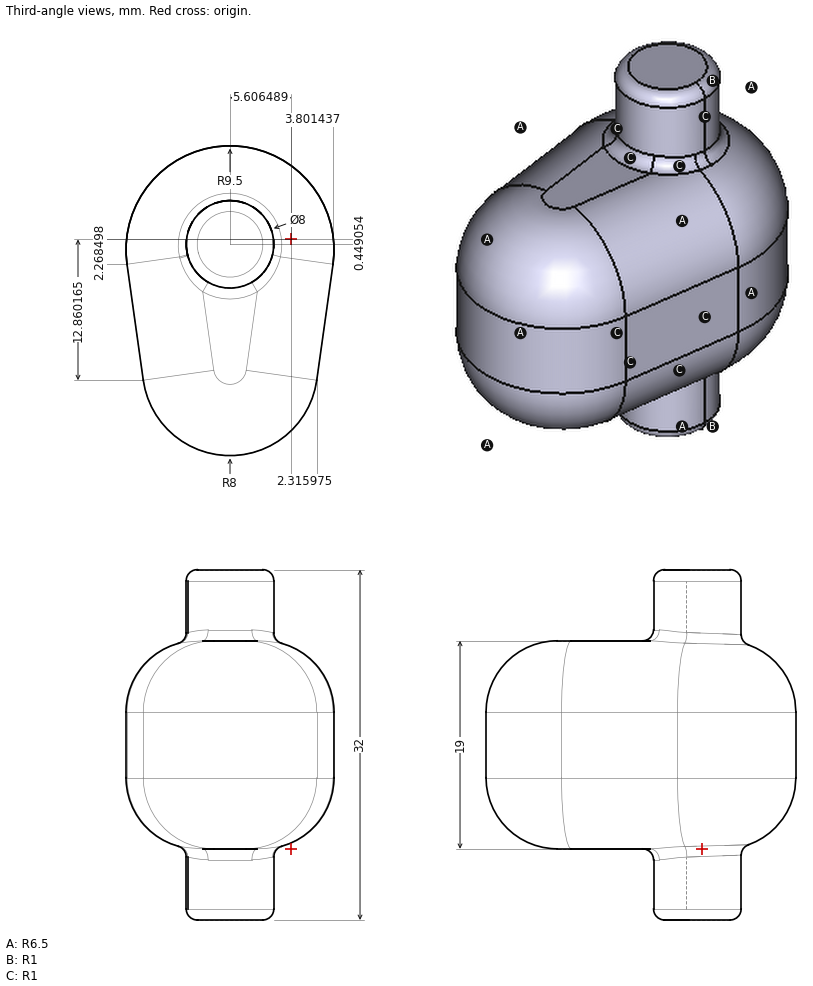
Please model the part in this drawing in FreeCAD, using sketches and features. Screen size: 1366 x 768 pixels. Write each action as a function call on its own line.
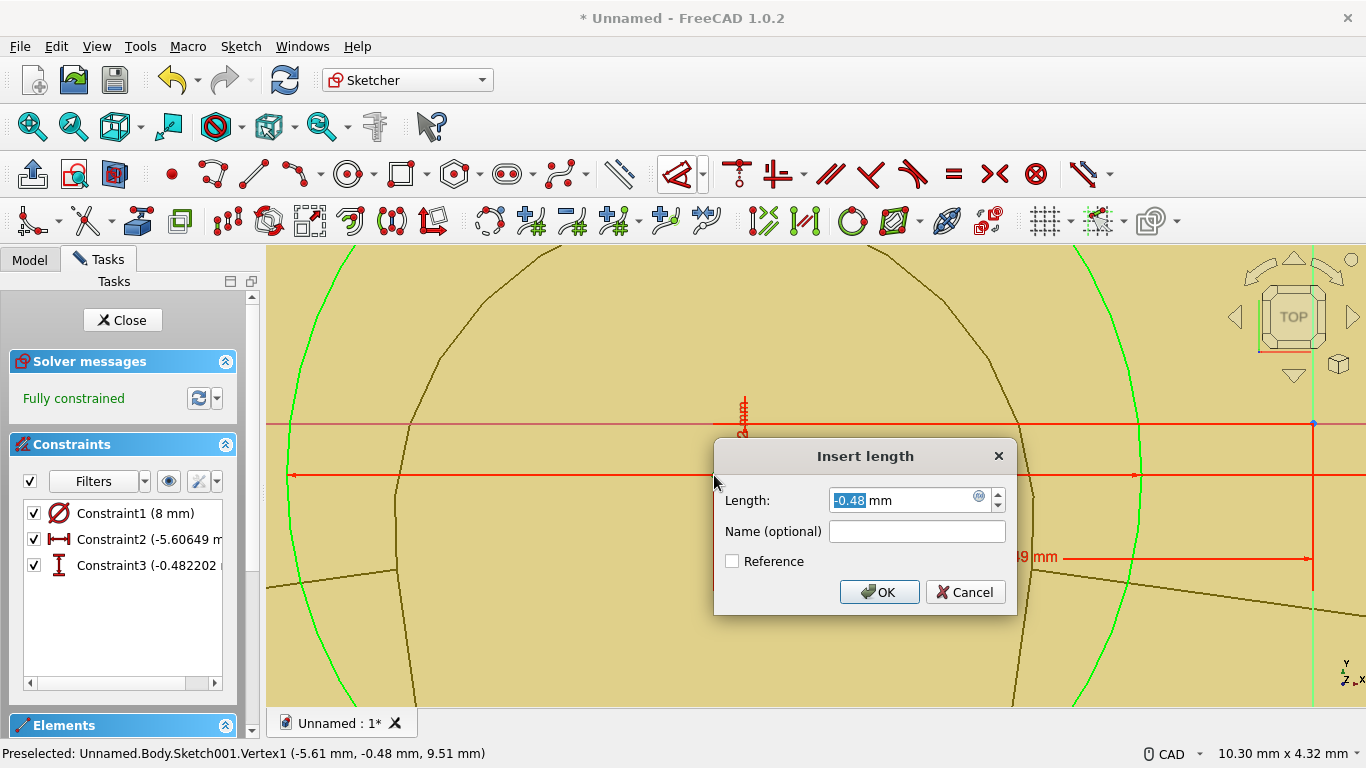
text(-0.449054)
key(Return)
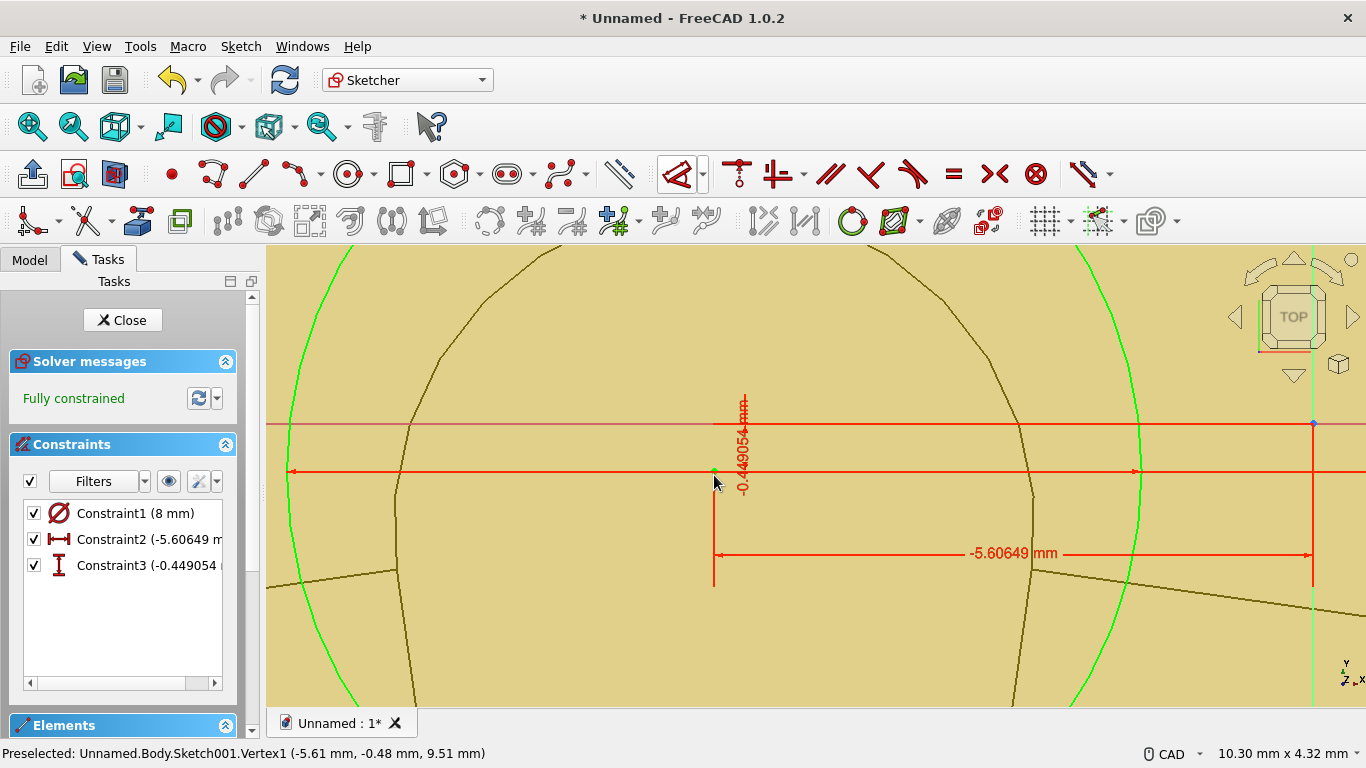
click(123, 320)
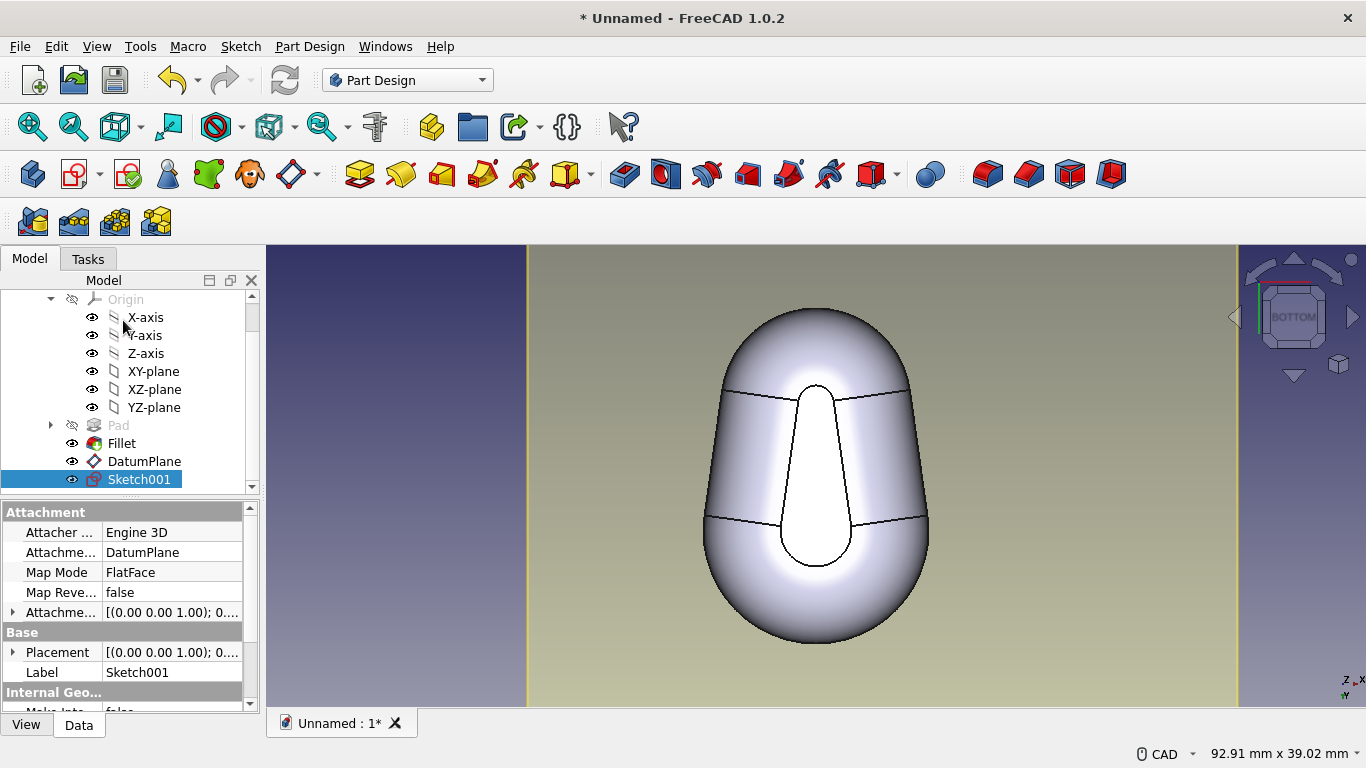
click(360, 174)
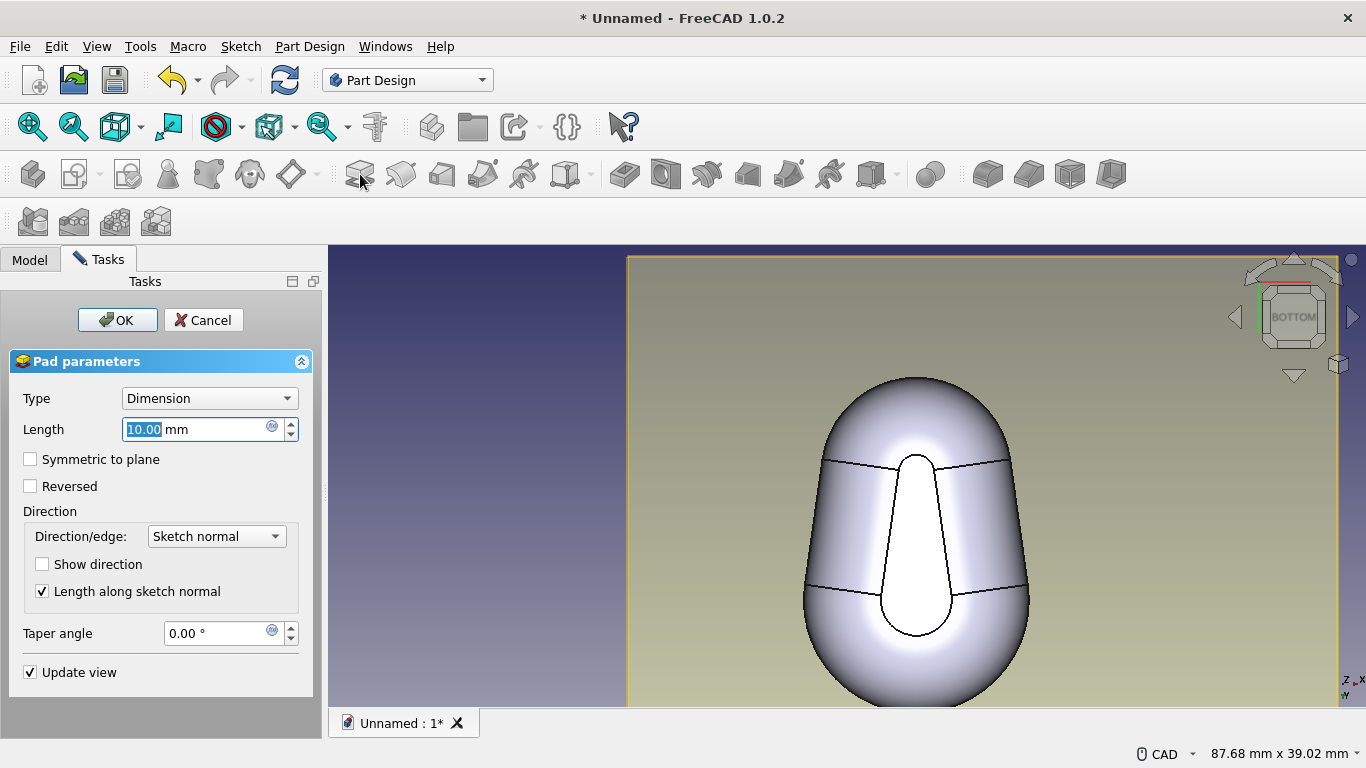
text(32)
key(Tab)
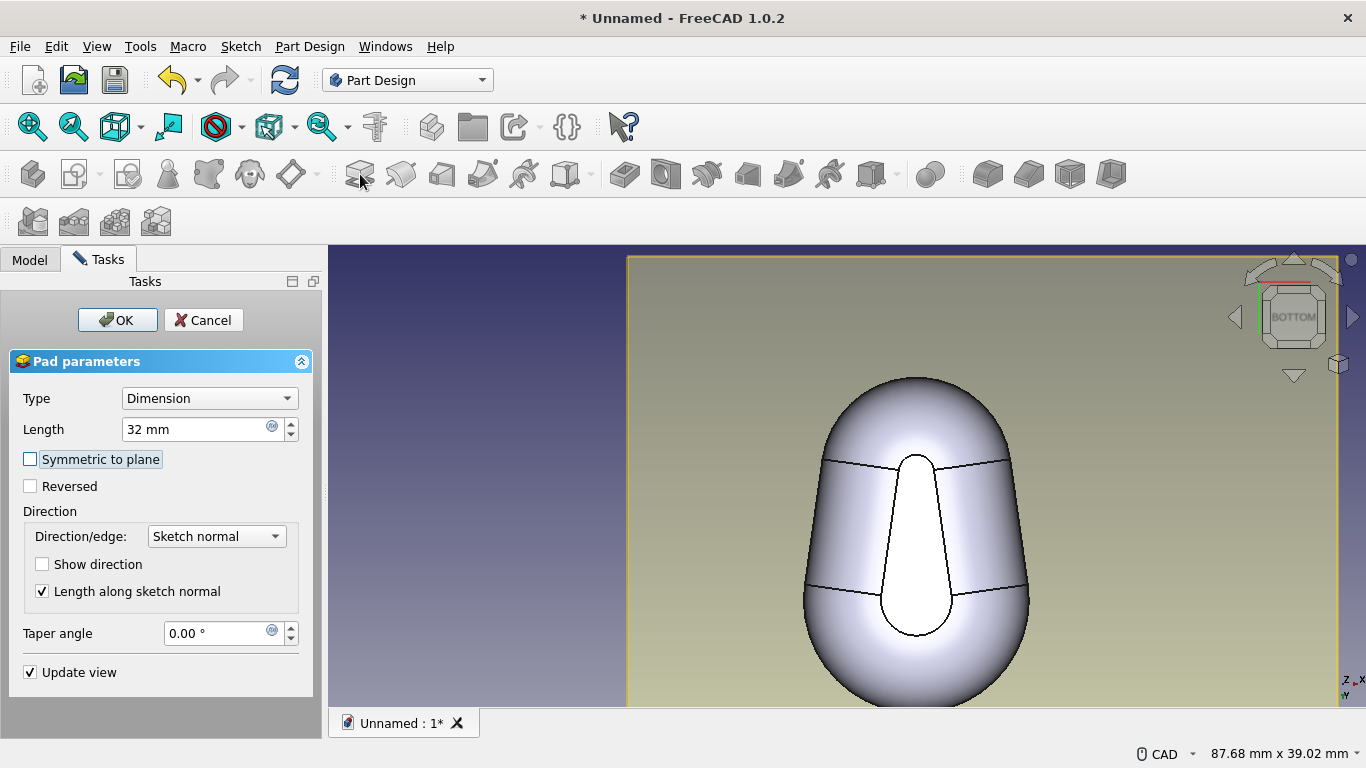
click(31, 459)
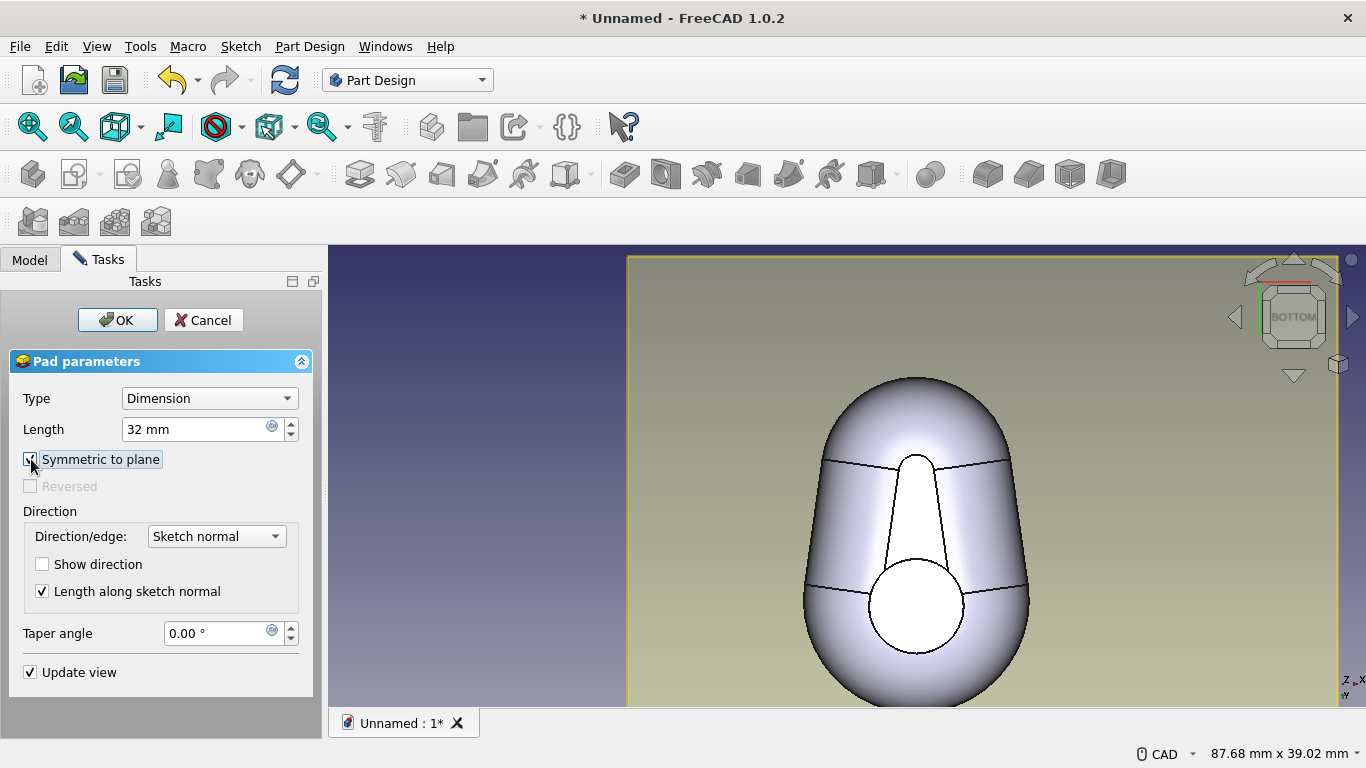
click(118, 320)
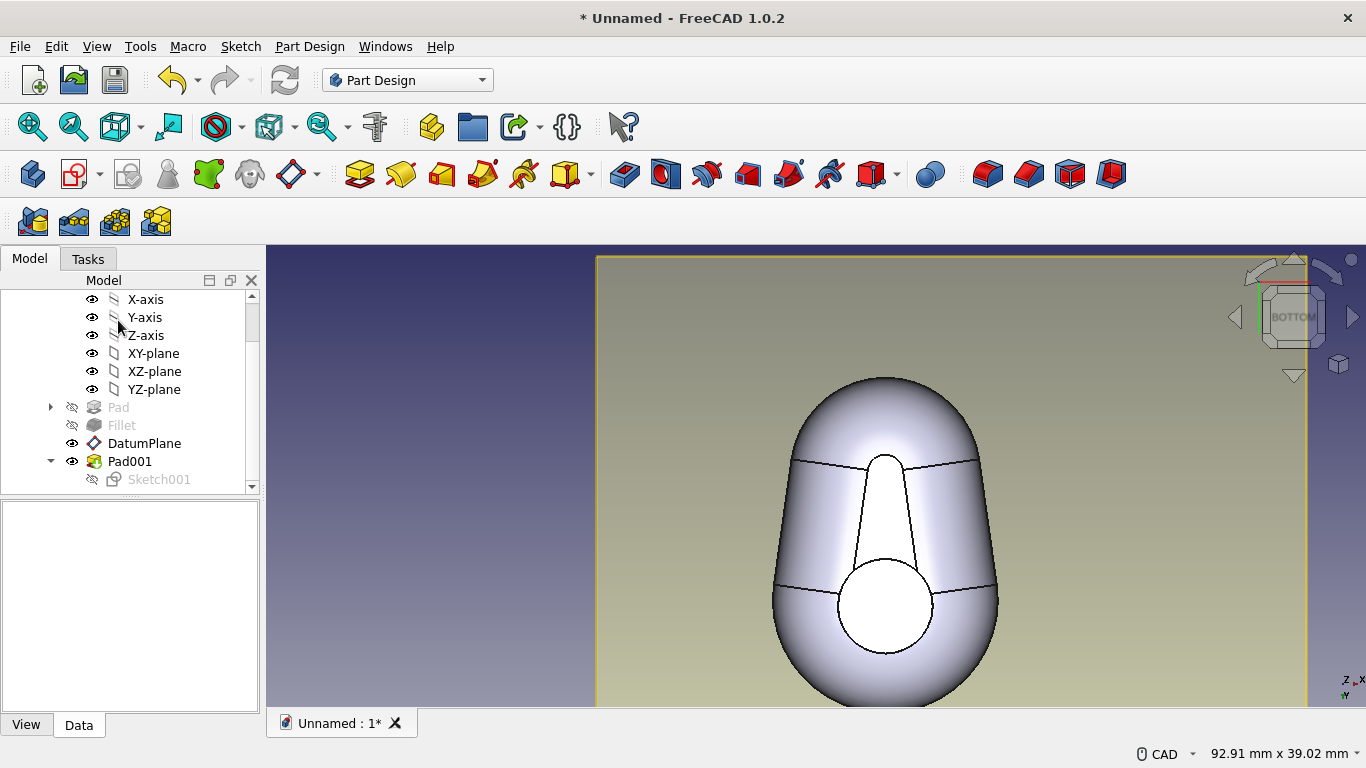
click(117, 443)
key(space)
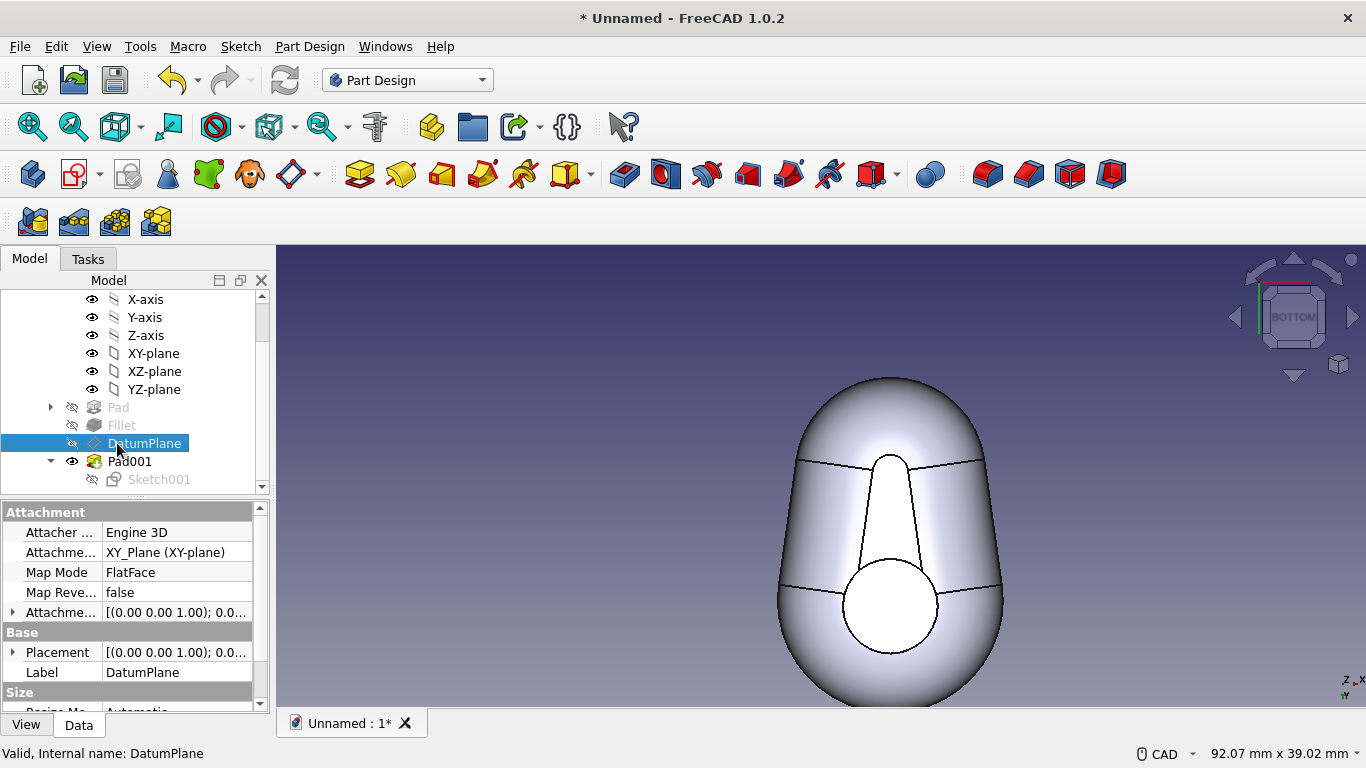
key(v)
key(f)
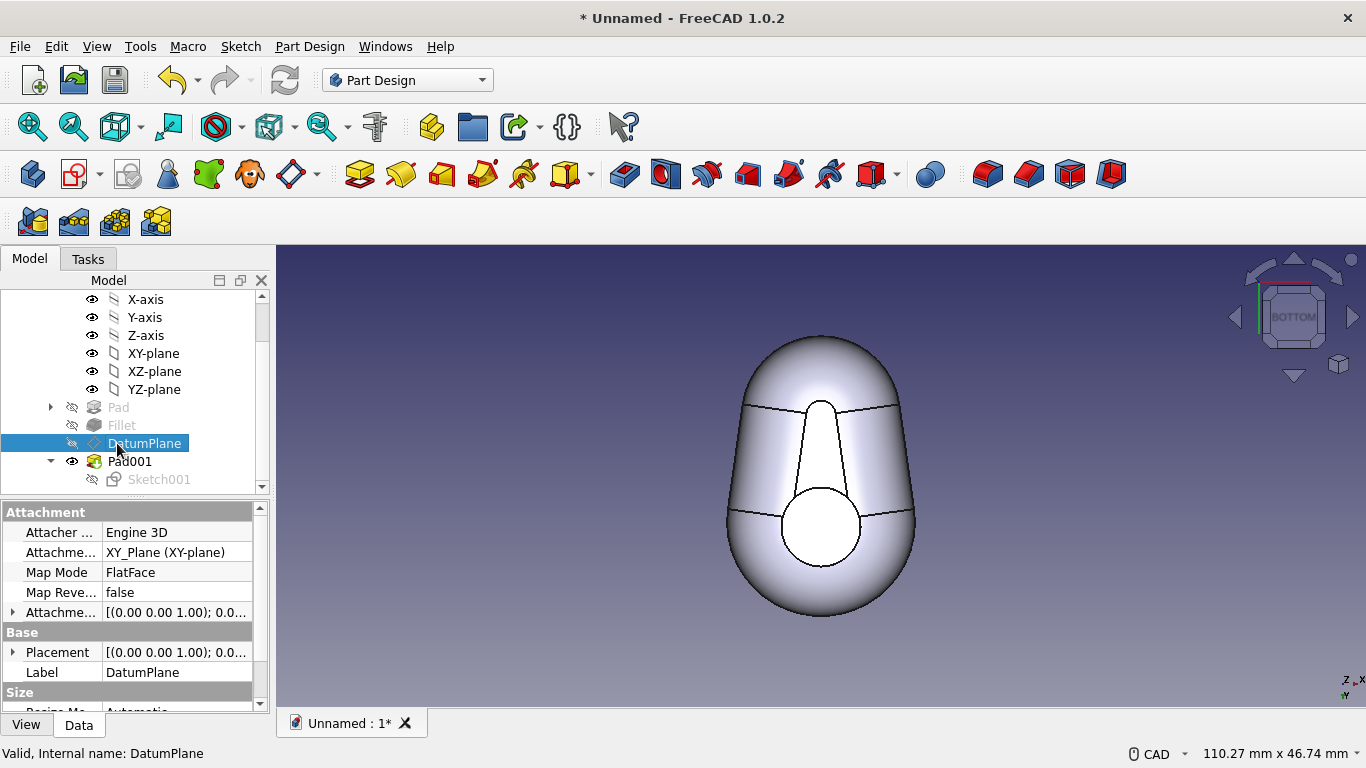
click(781, 526)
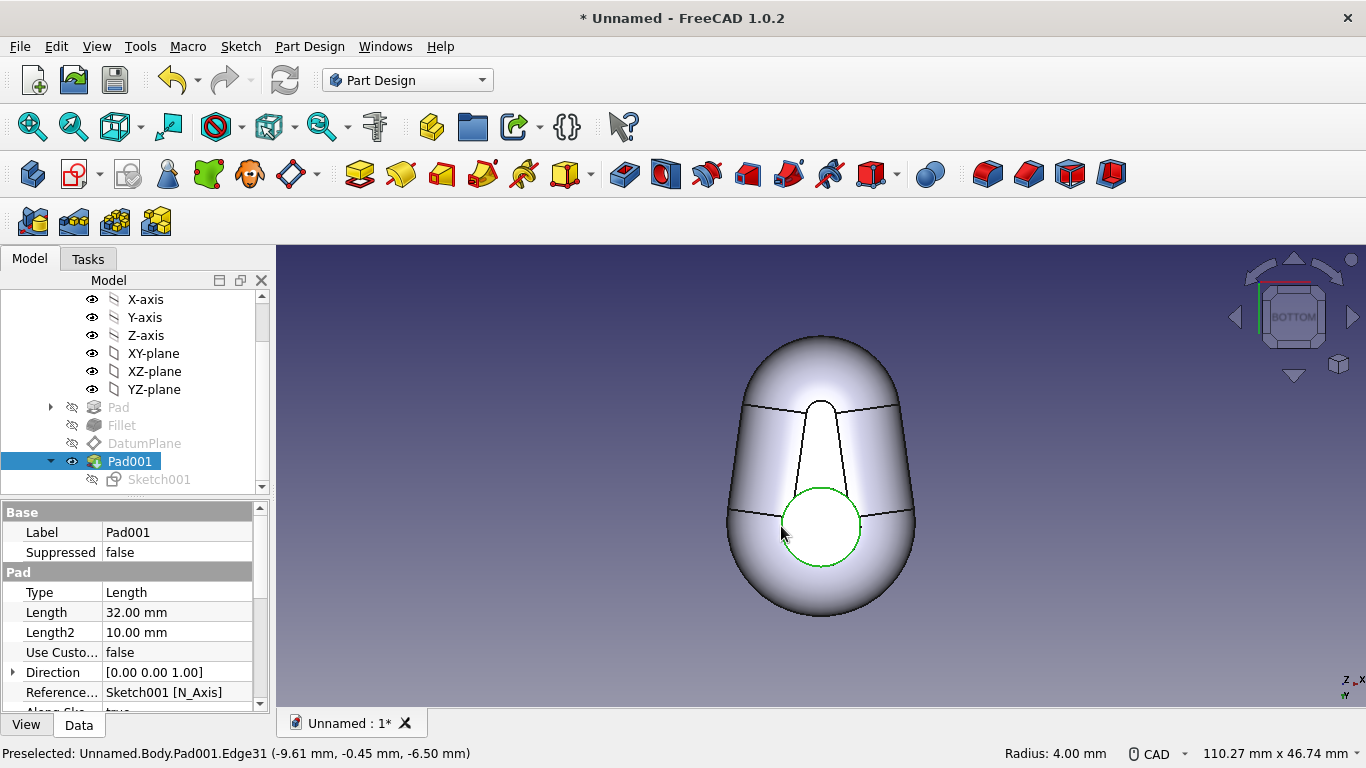
key(0)